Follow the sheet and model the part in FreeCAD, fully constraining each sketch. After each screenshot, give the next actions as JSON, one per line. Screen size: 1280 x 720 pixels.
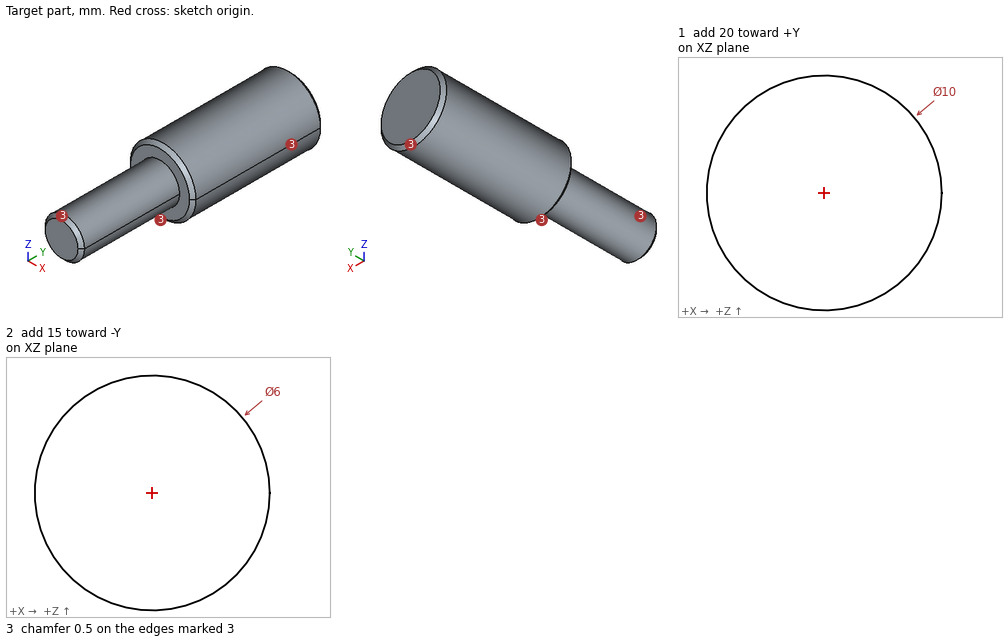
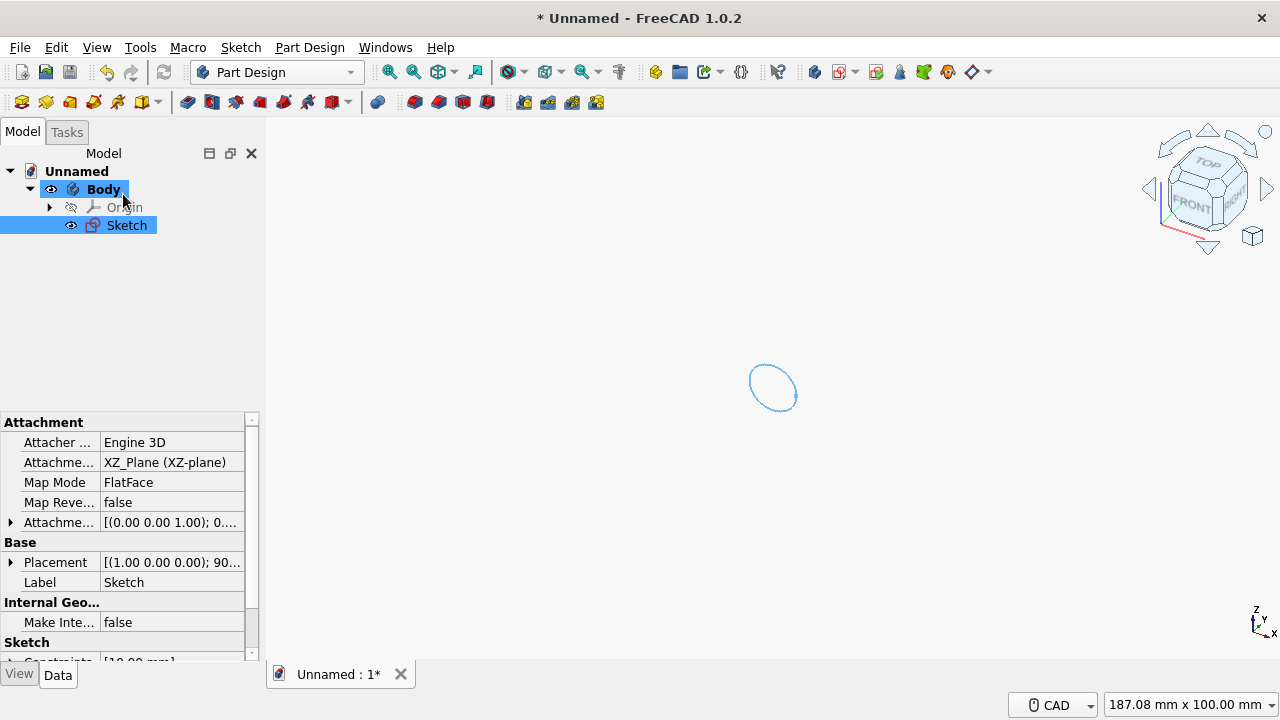
{"action": "left_click", "coordinate": [22, 102]}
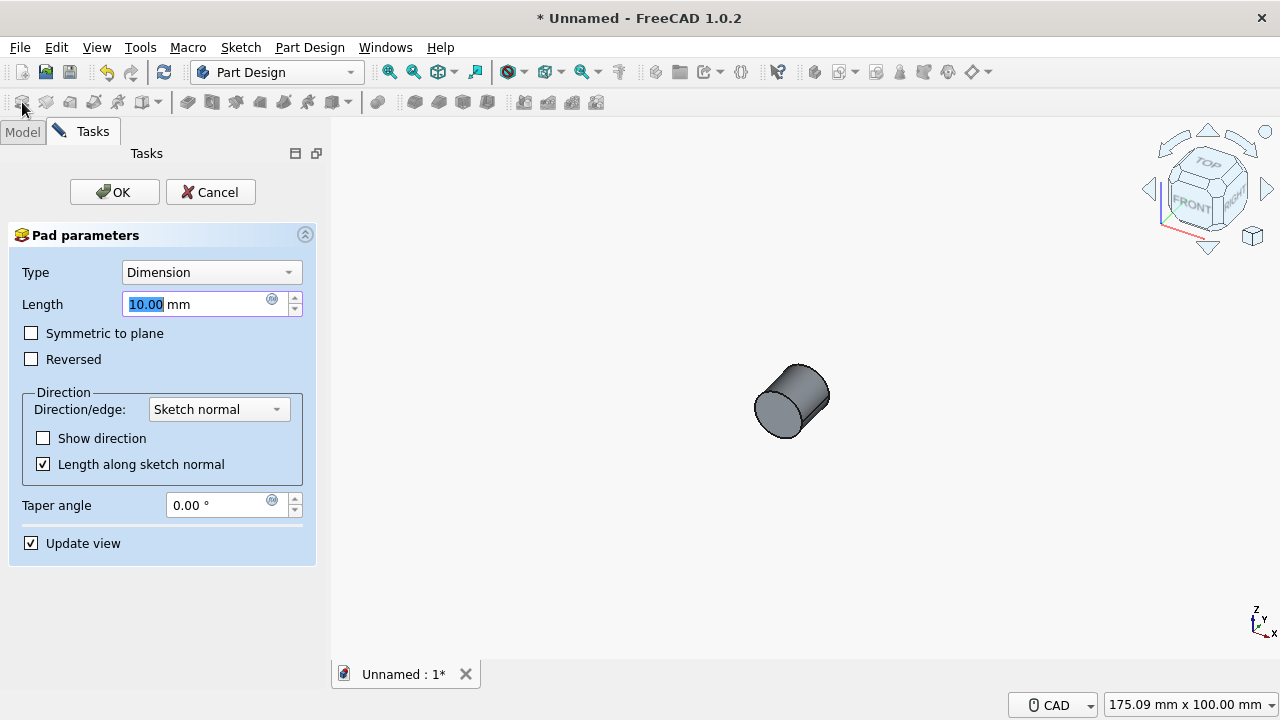
{"action": "type", "text": "20"}
{"action": "key", "text": "Tab"}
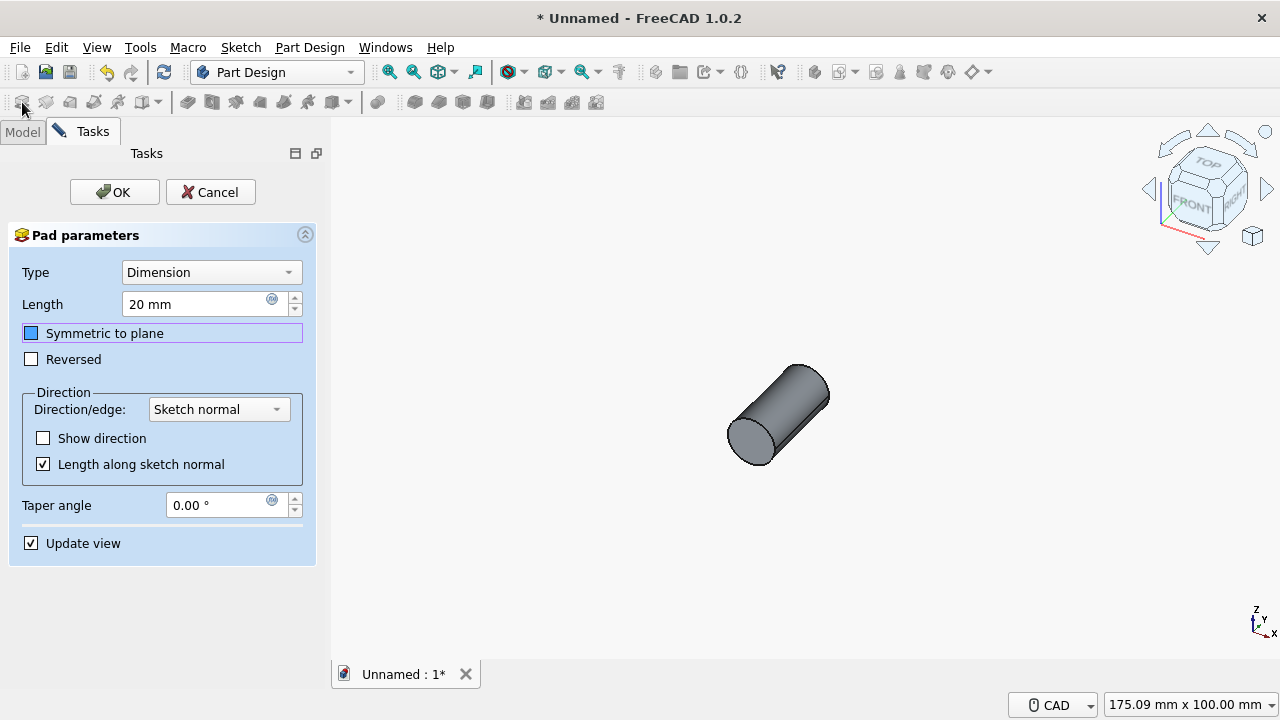
{"action": "left_click", "coordinate": [30, 359]}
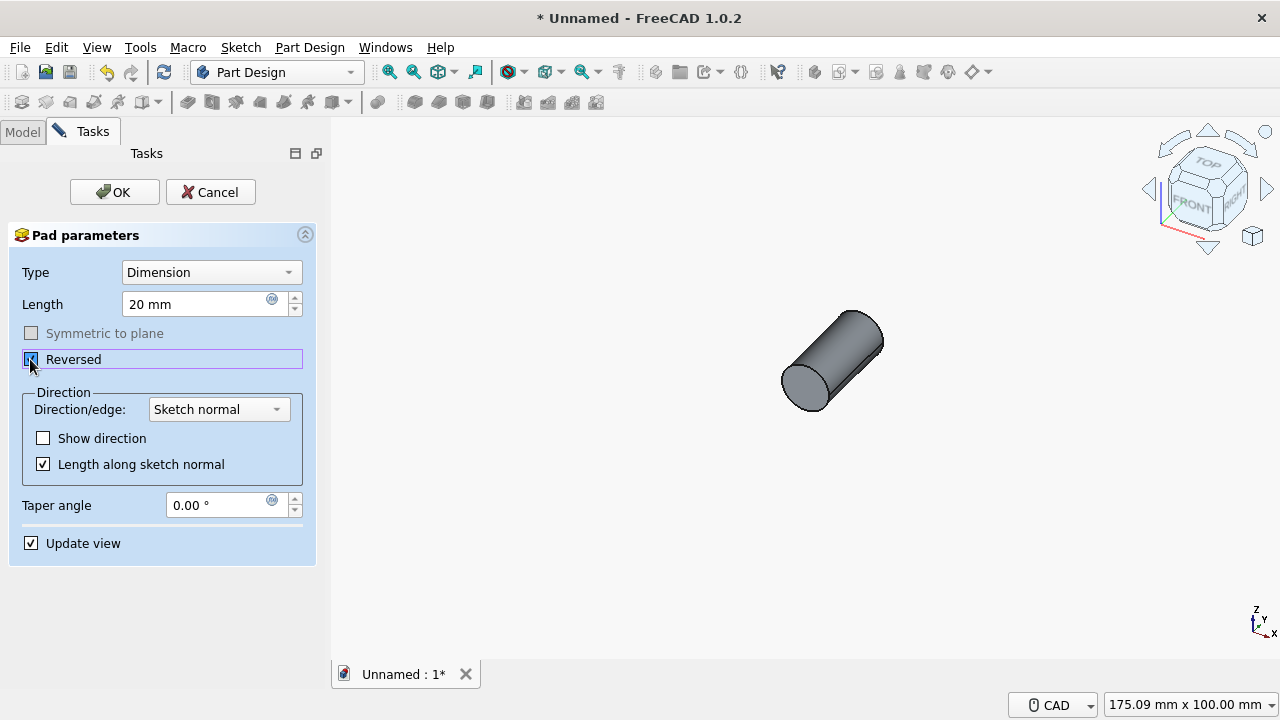
{"action": "left_click", "coordinate": [115, 192]}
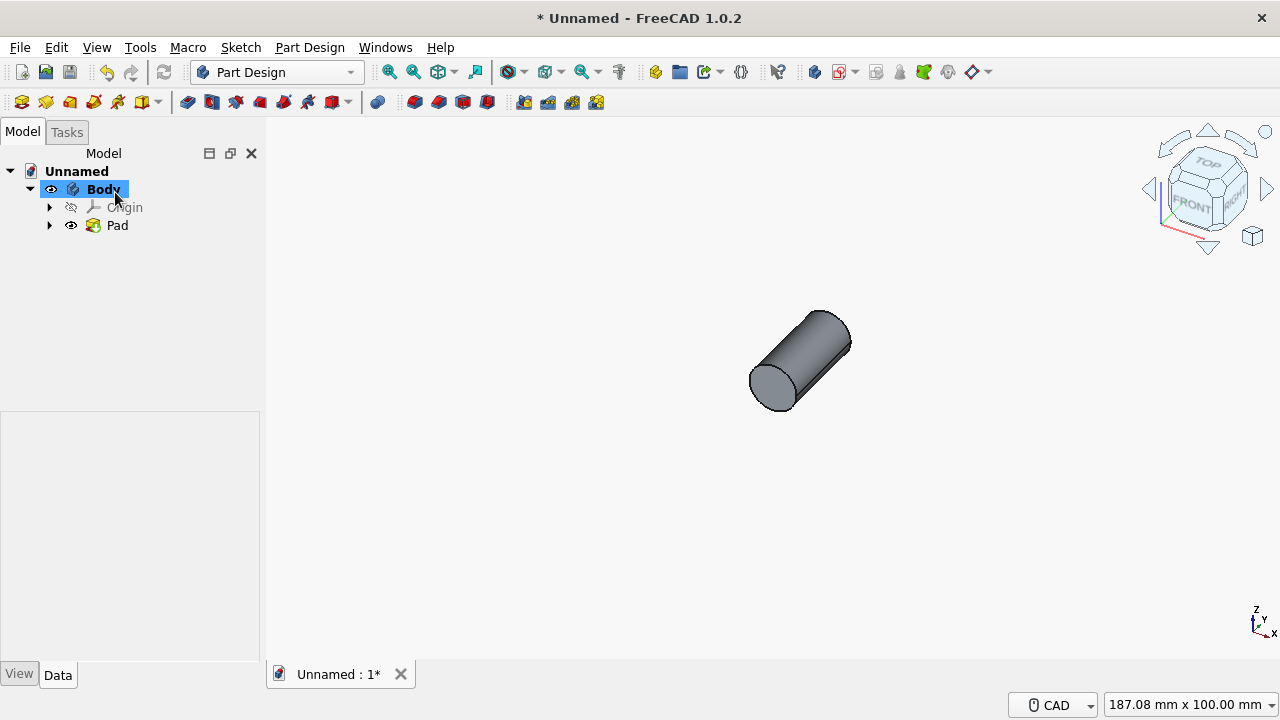
{"action": "left_click", "coordinate": [390, 72]}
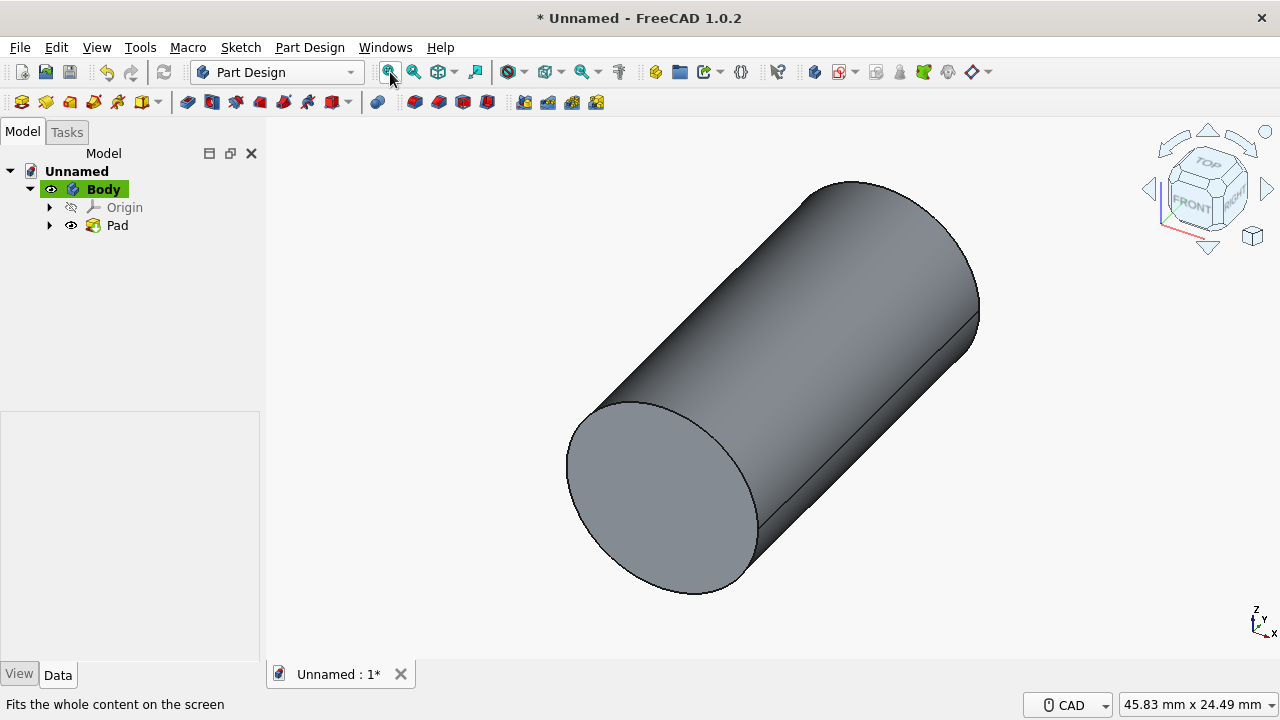
{"action": "left_click", "coordinate": [840, 72]}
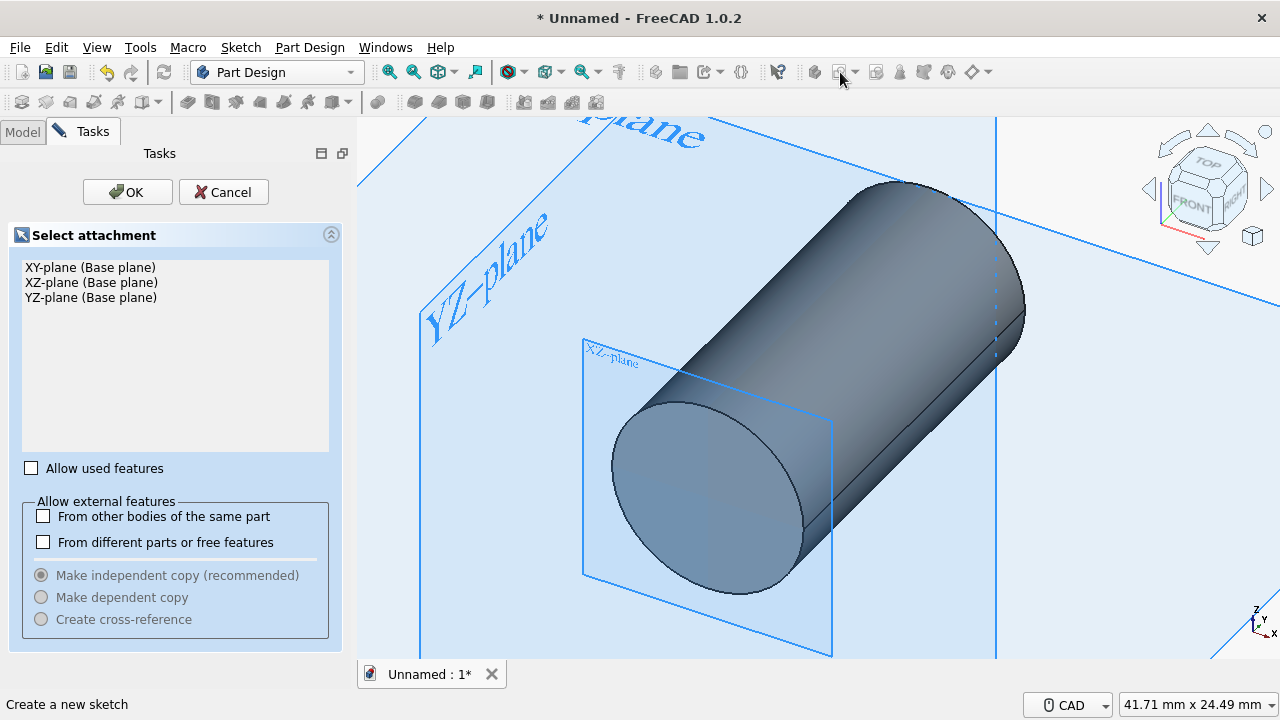
{"action": "left_click", "coordinate": [82, 282]}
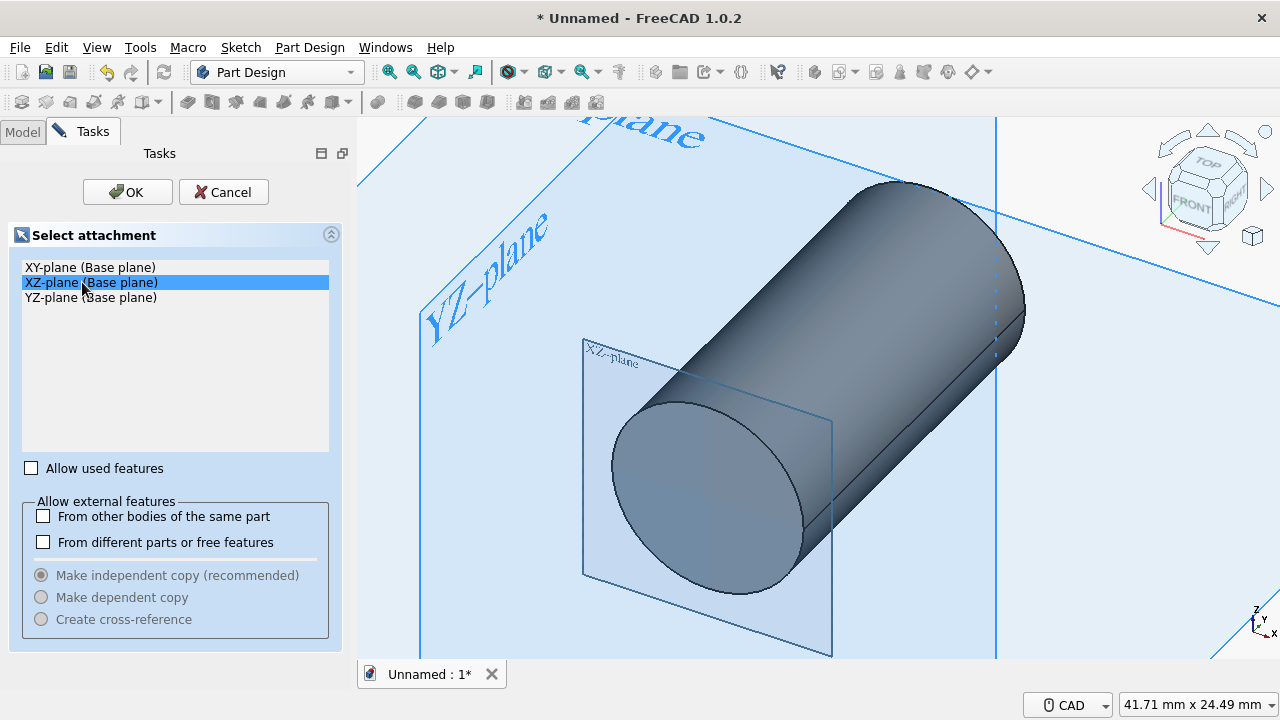
{"action": "left_click", "coordinate": [128, 192]}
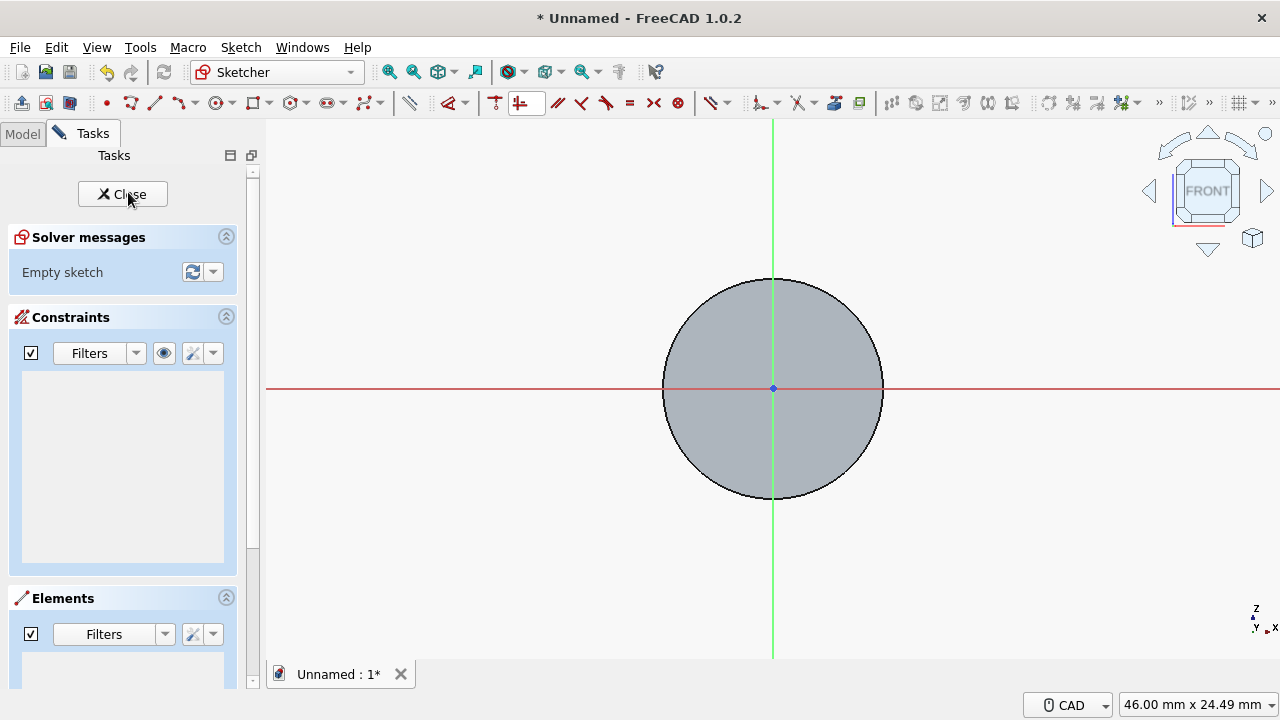
{"action": "scroll", "coordinate": [813, 389], "scroll_direction": "up", "scroll_amount": 5}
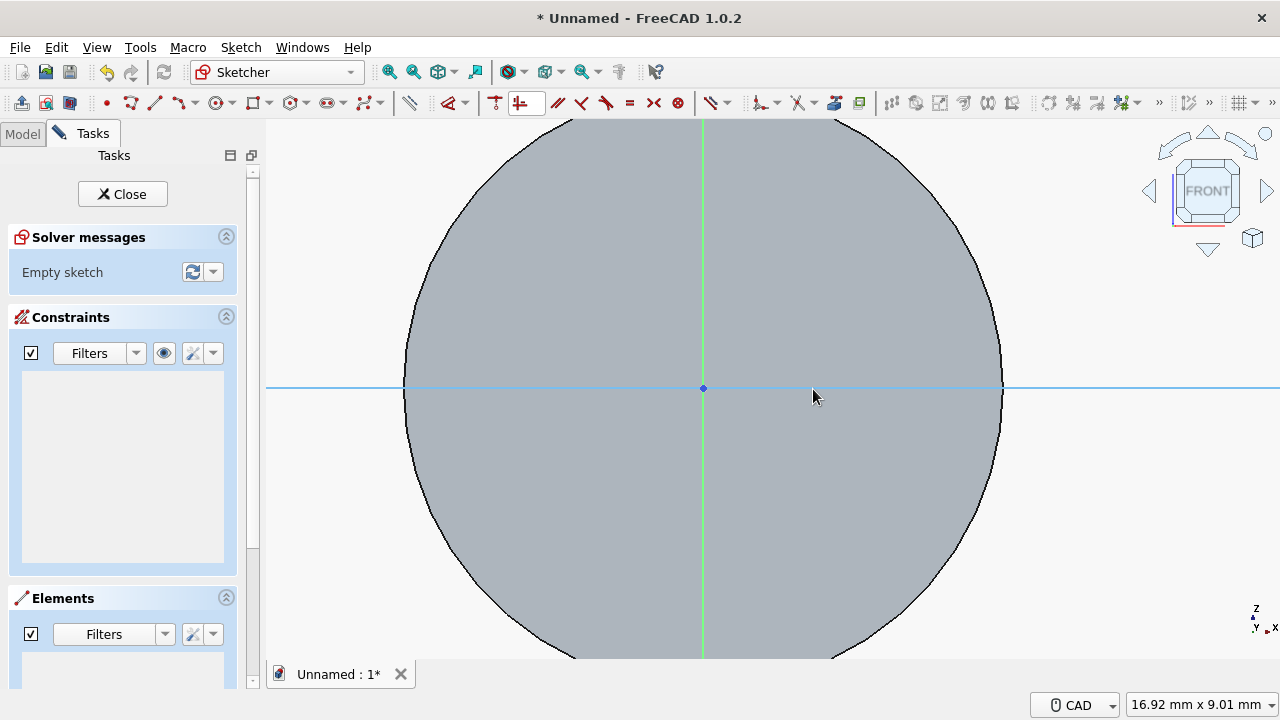
{"action": "left_click", "coordinate": [216, 104]}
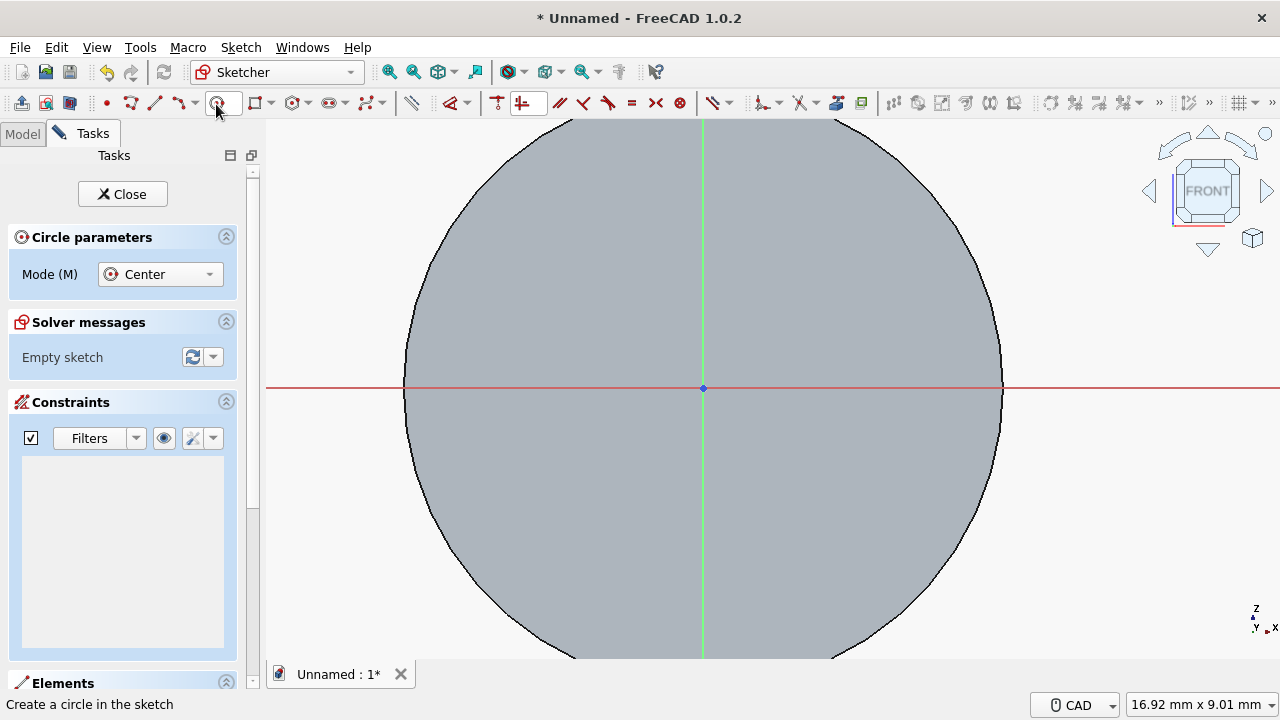
{"action": "left_click", "coordinate": [703, 388]}
{"action": "left_click", "coordinate": [830, 261]}
{"action": "key", "text": "Escape"}